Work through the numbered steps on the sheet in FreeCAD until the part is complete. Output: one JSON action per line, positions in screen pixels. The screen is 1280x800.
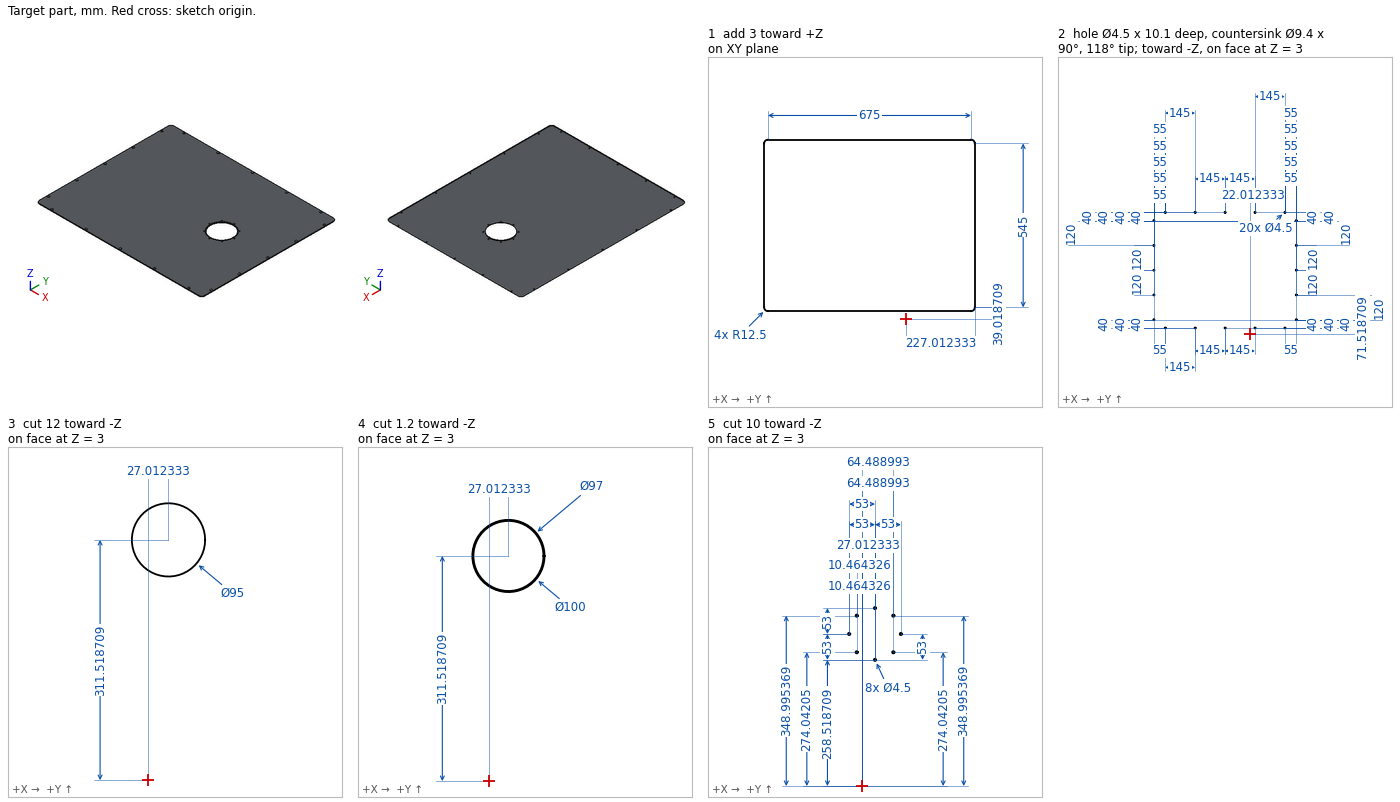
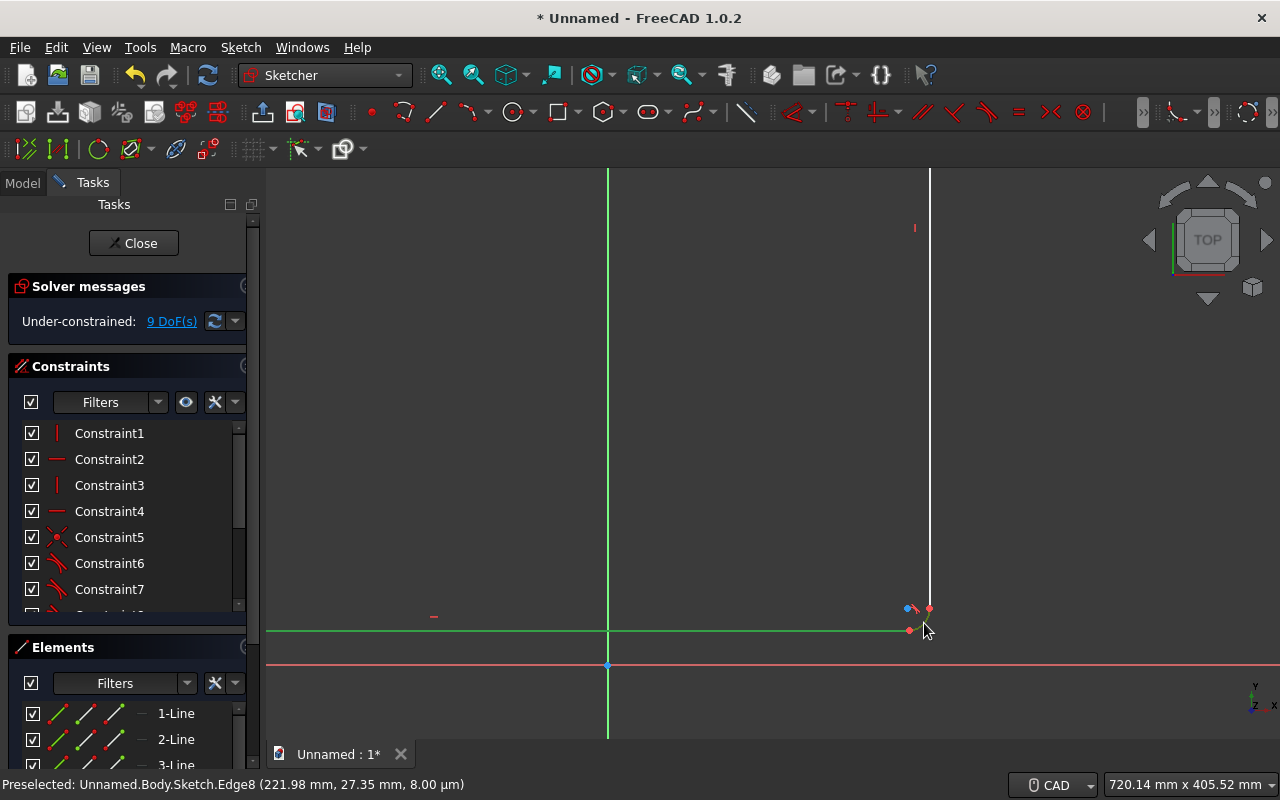
{"action": "left_click", "coordinate": [988, 112]}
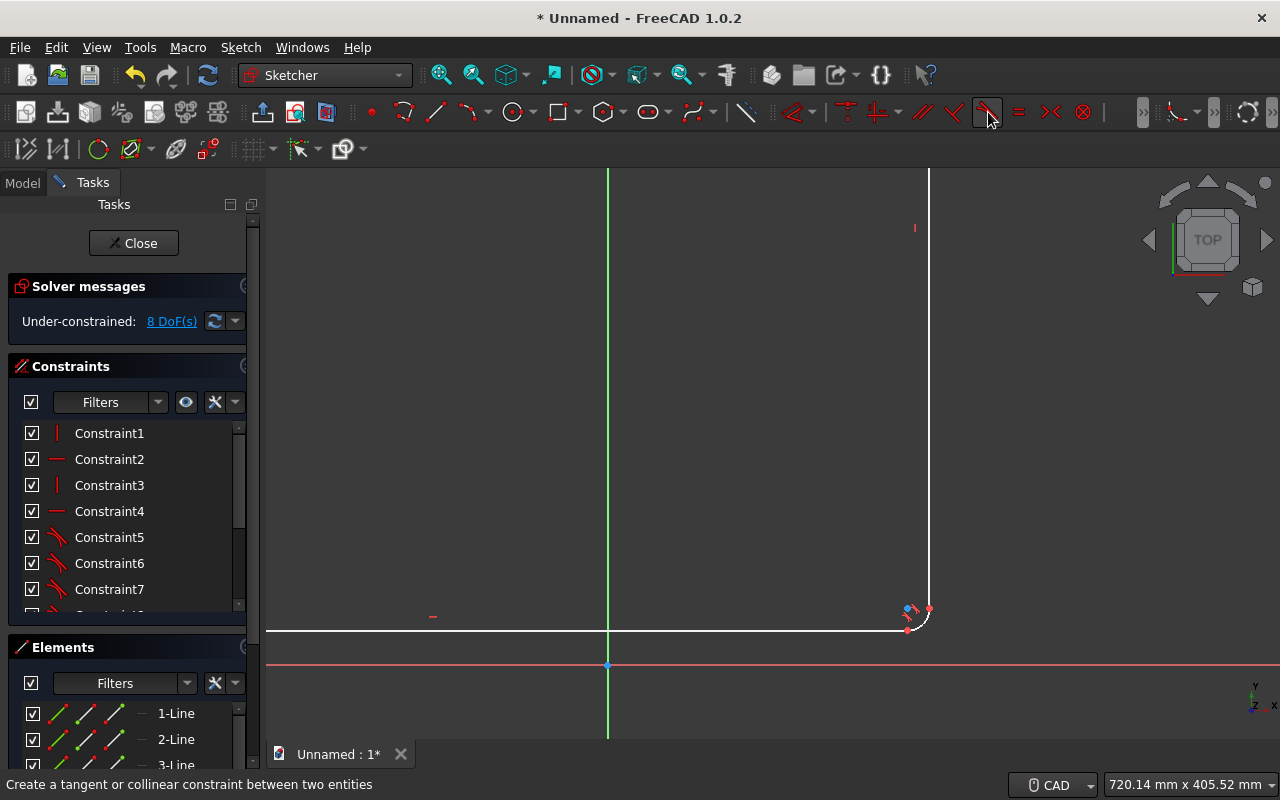
{"action": "scroll", "coordinate": [925, 623], "scroll_direction": "down", "scroll_amount": 4}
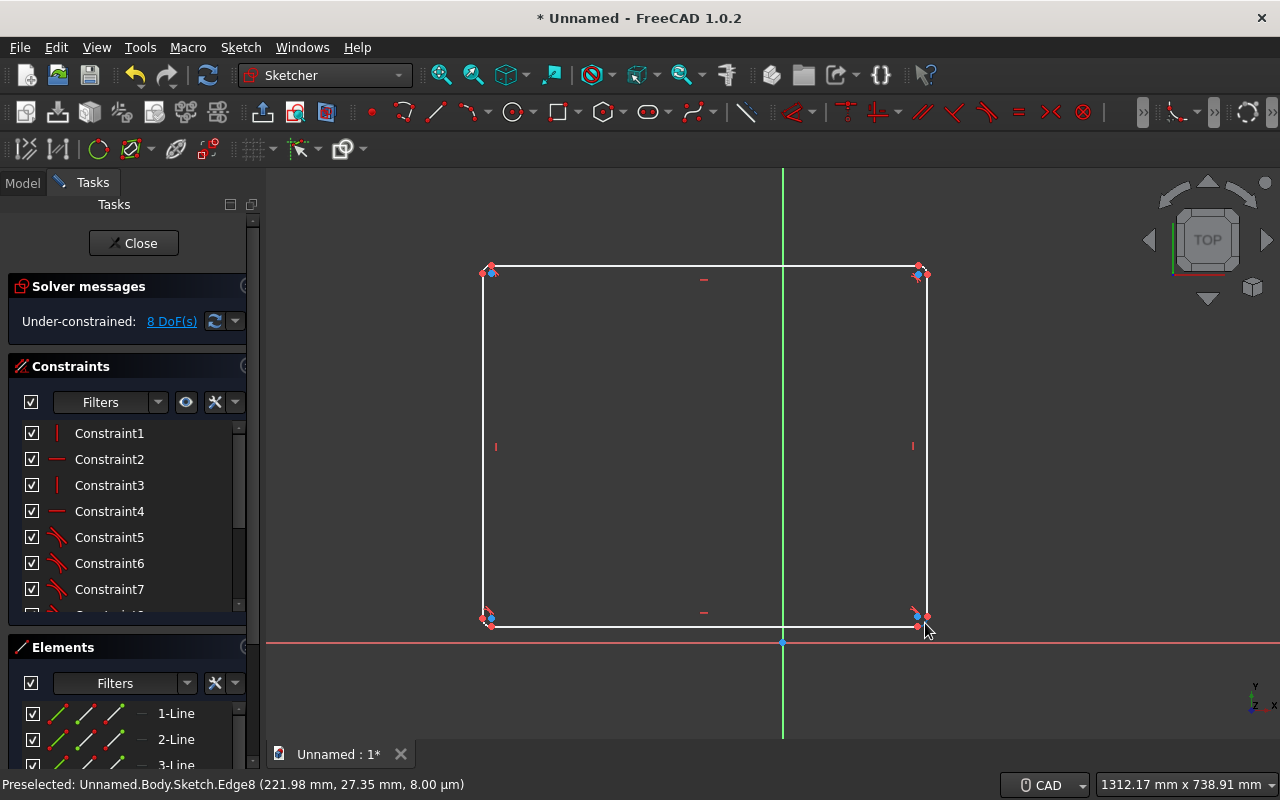
{"action": "scroll", "coordinate": [926, 271], "scroll_direction": "up", "scroll_amount": 6}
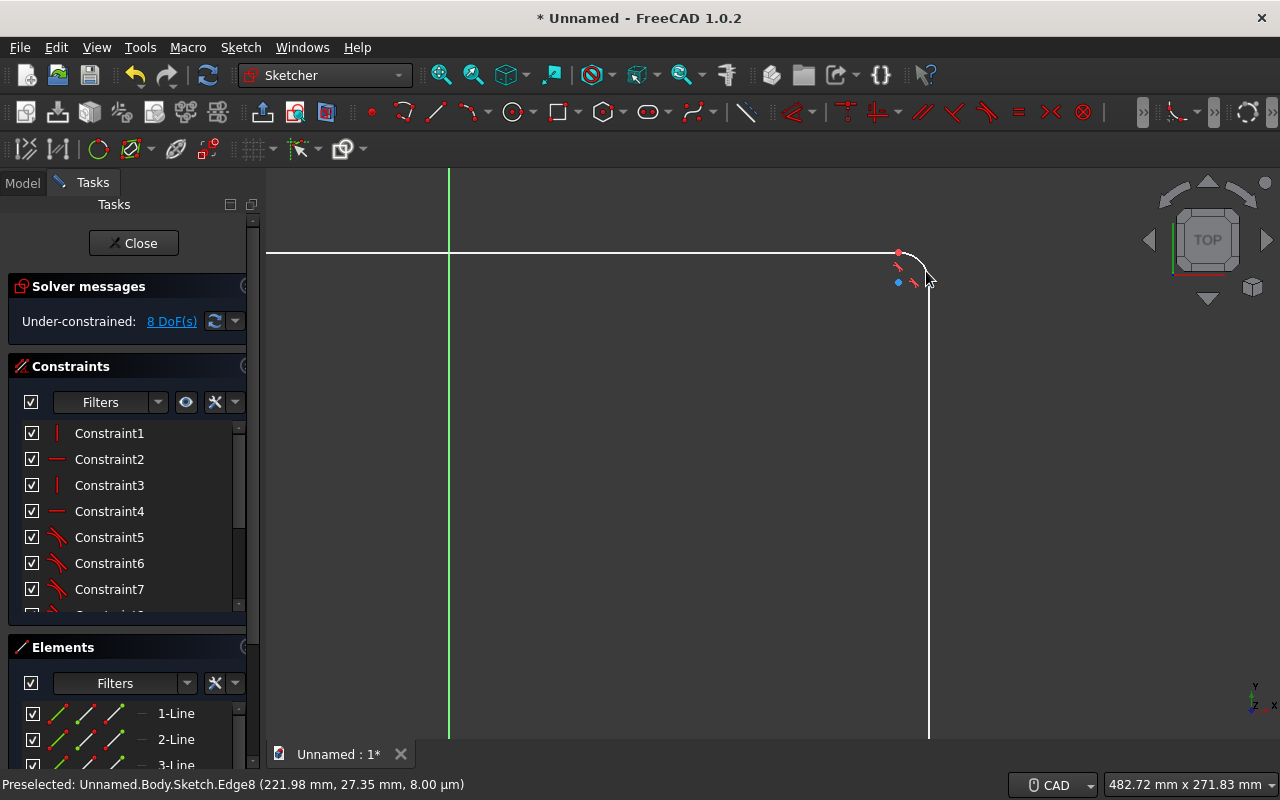
{"action": "left_click", "coordinate": [926, 269]}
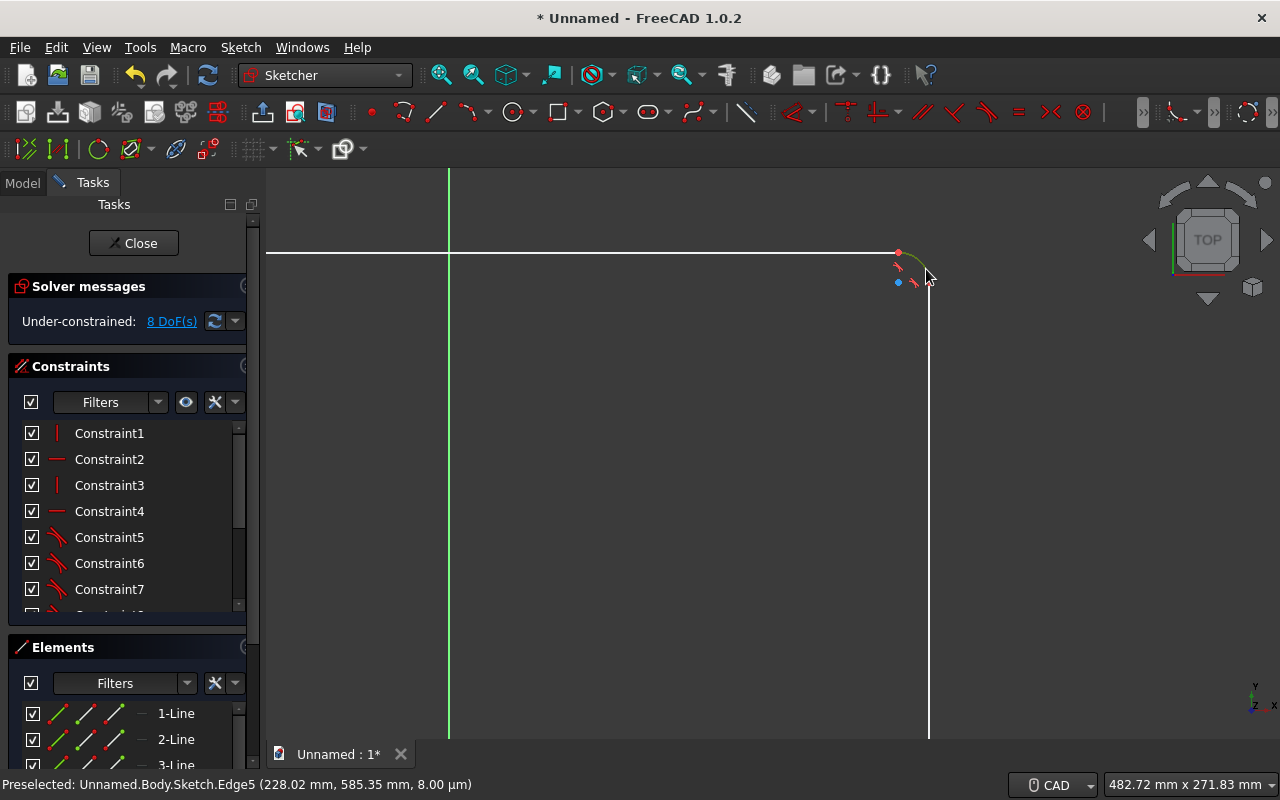
{"action": "scroll", "coordinate": [926, 271], "scroll_direction": "down", "scroll_amount": 6}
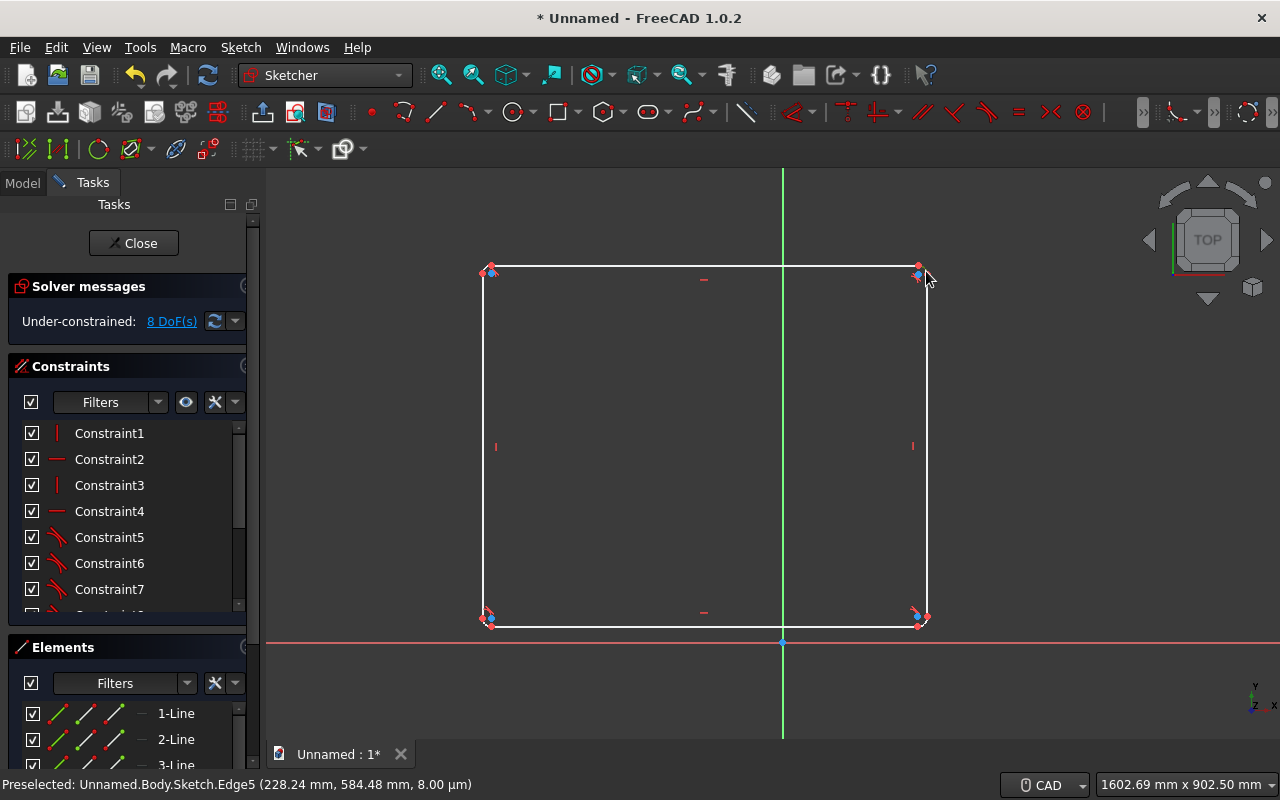
{"action": "scroll", "coordinate": [487, 267], "scroll_direction": "up", "scroll_amount": 7}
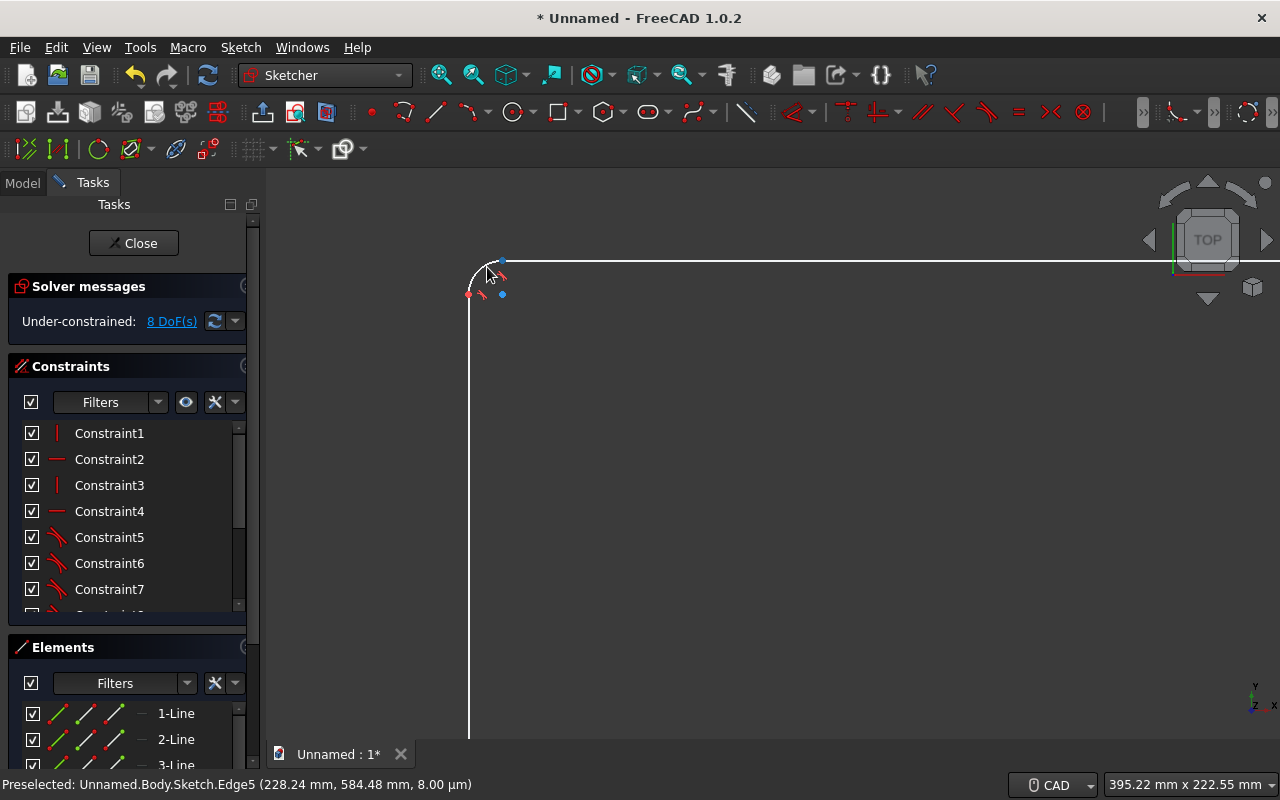
{"action": "left_click", "coordinate": [487, 264]}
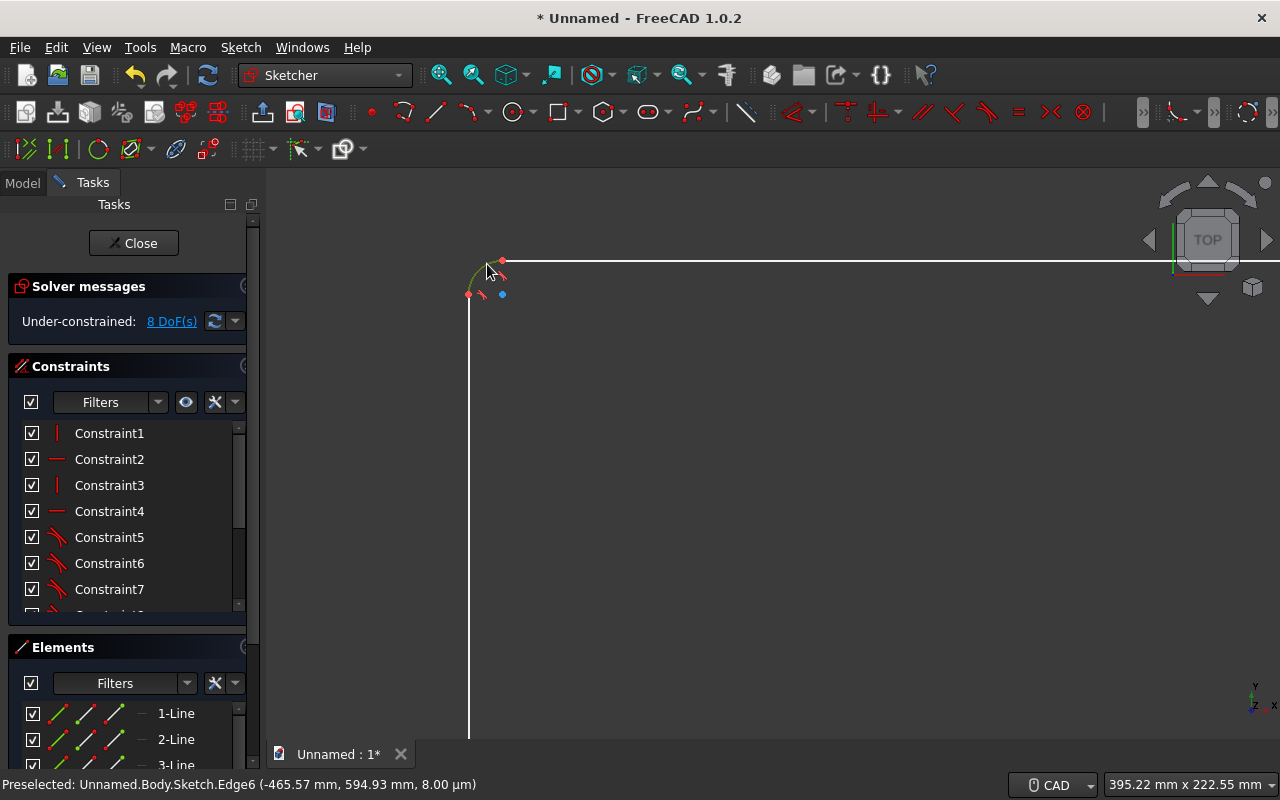
{"action": "scroll", "coordinate": [487, 267], "scroll_direction": "down", "scroll_amount": 7}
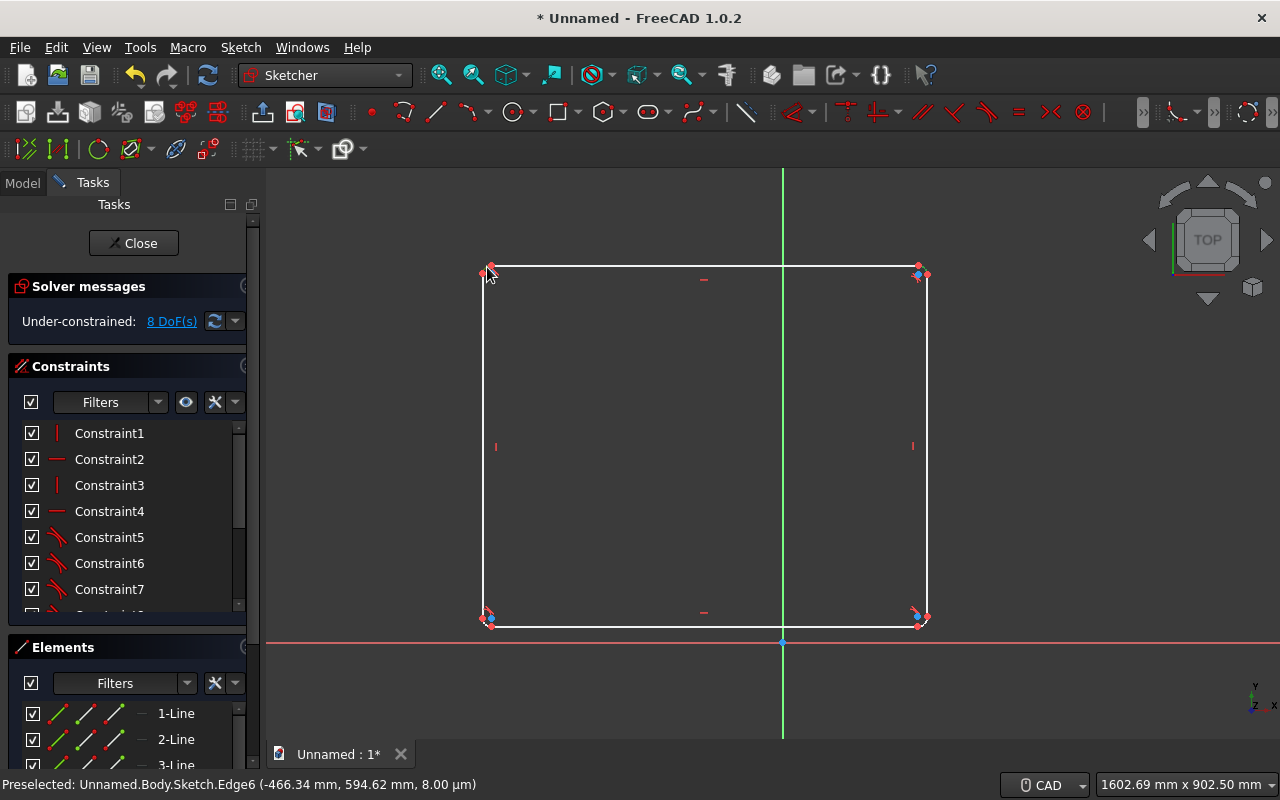
{"action": "scroll", "coordinate": [484, 622], "scroll_direction": "up", "scroll_amount": 7}